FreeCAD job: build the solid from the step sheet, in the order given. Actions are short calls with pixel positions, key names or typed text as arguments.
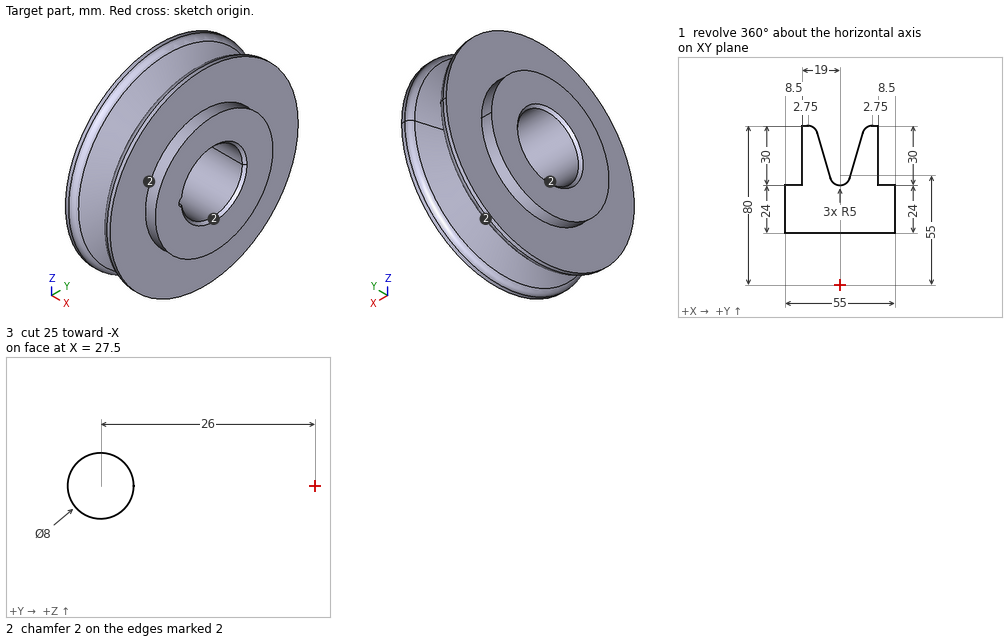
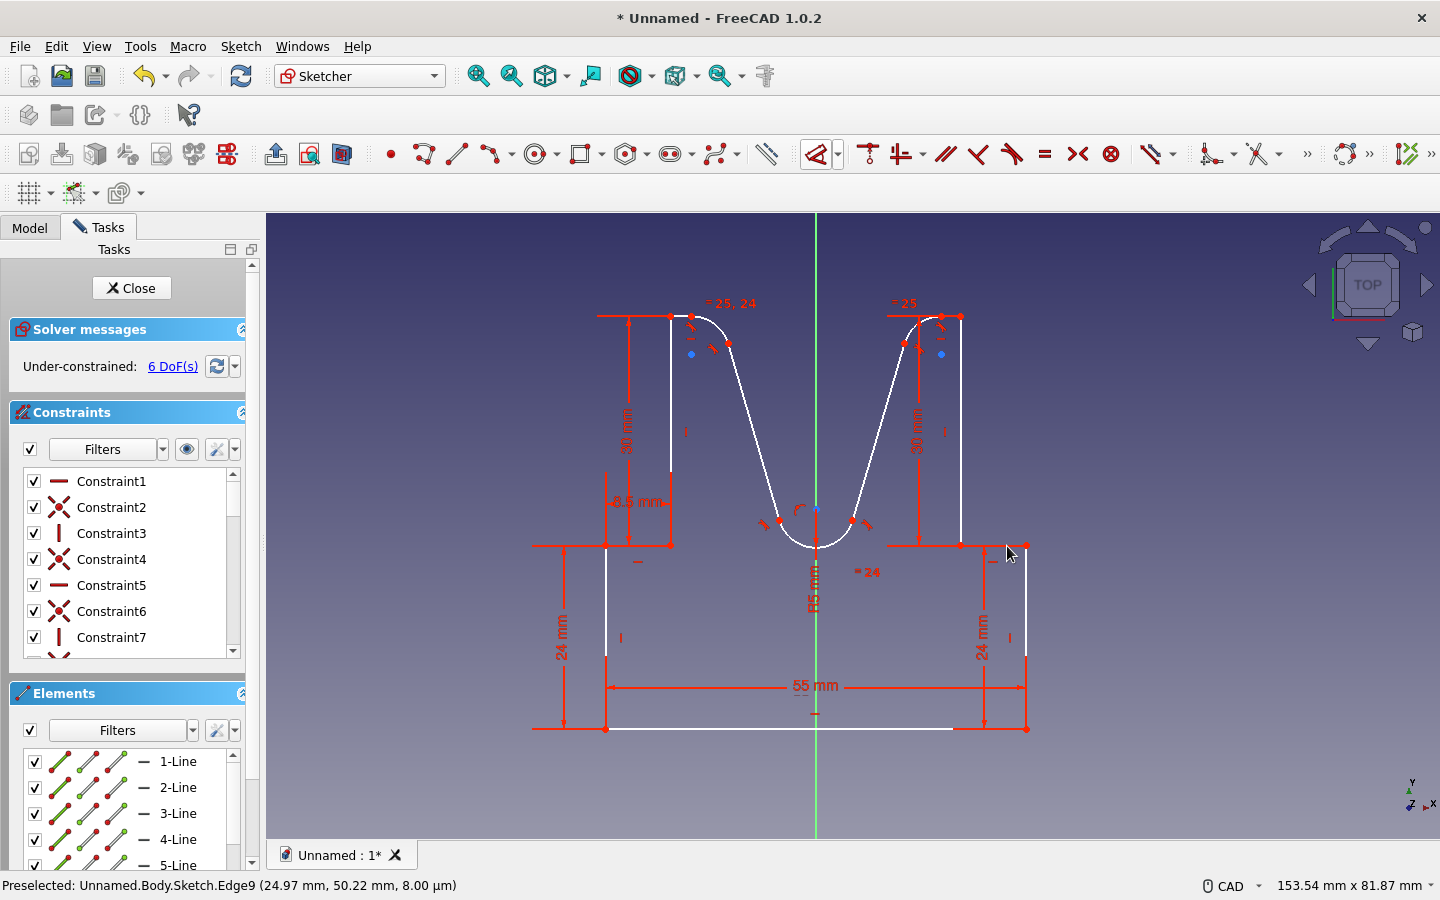
key(l)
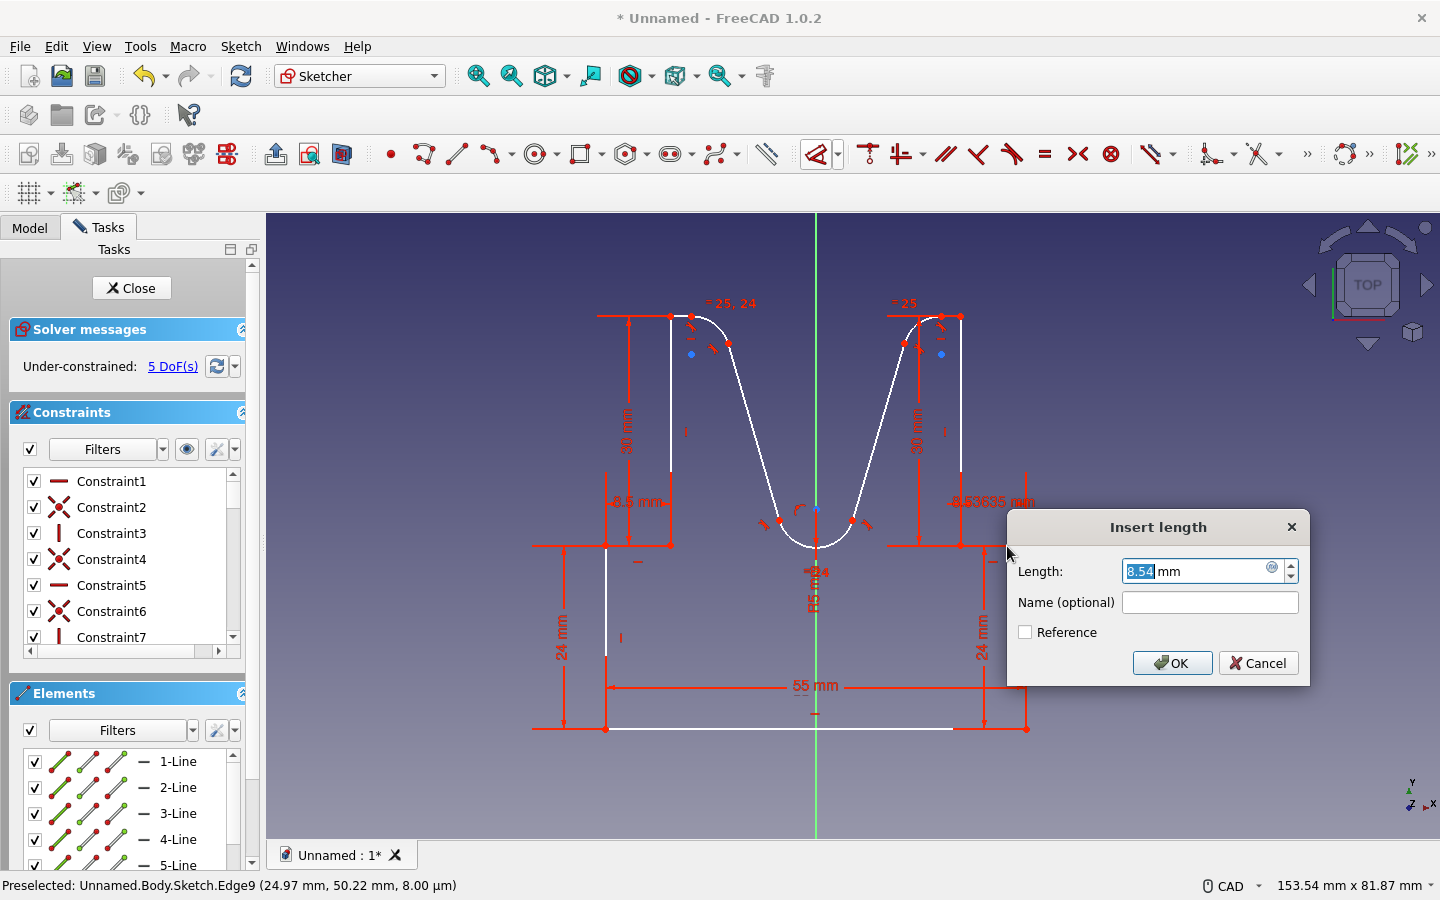
text(8.5)
key(Return)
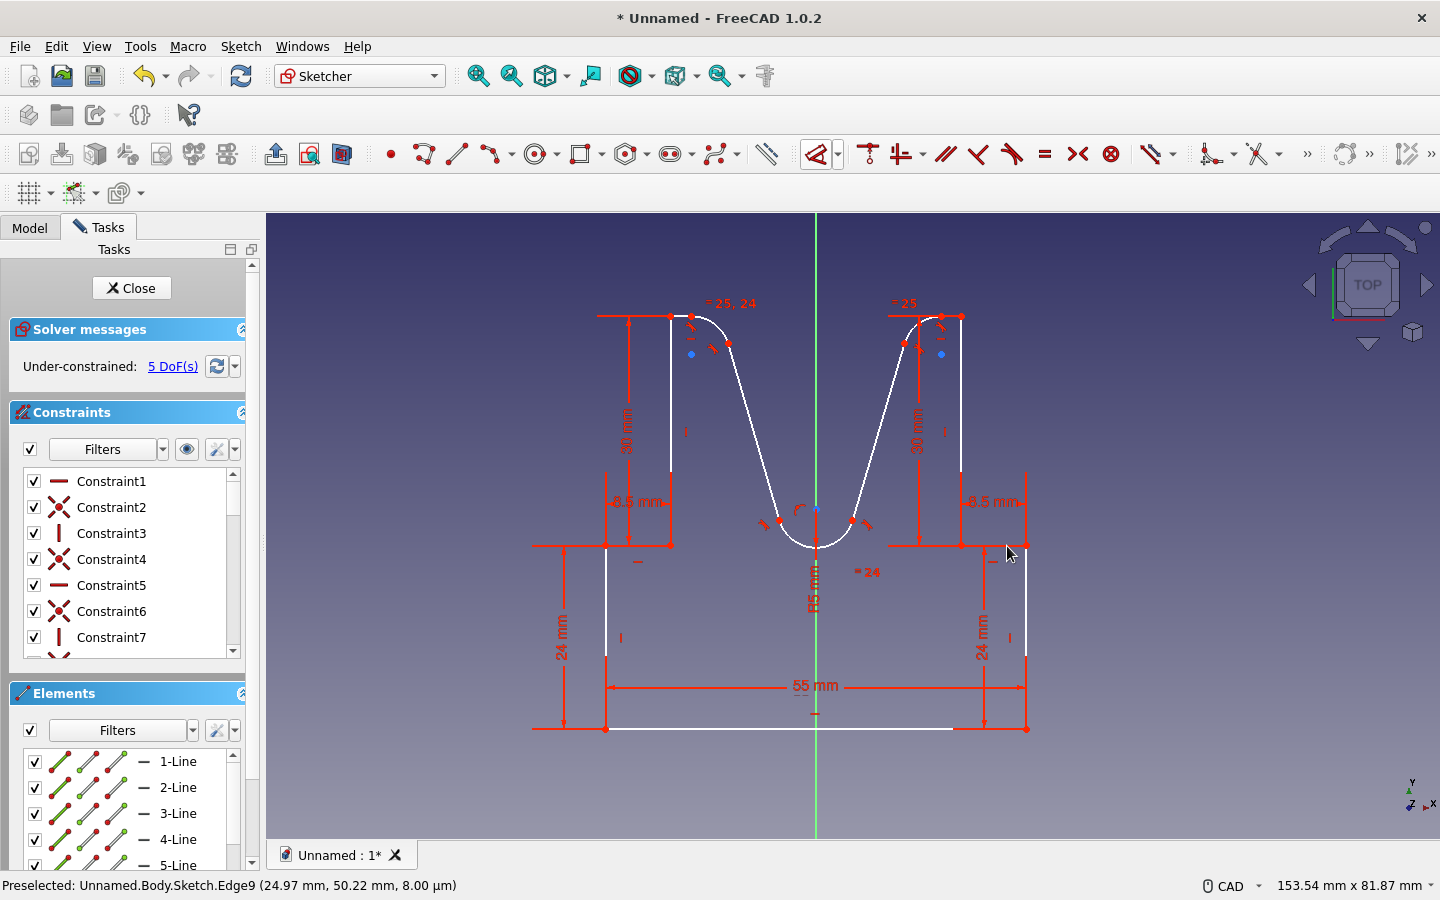
click(691, 316)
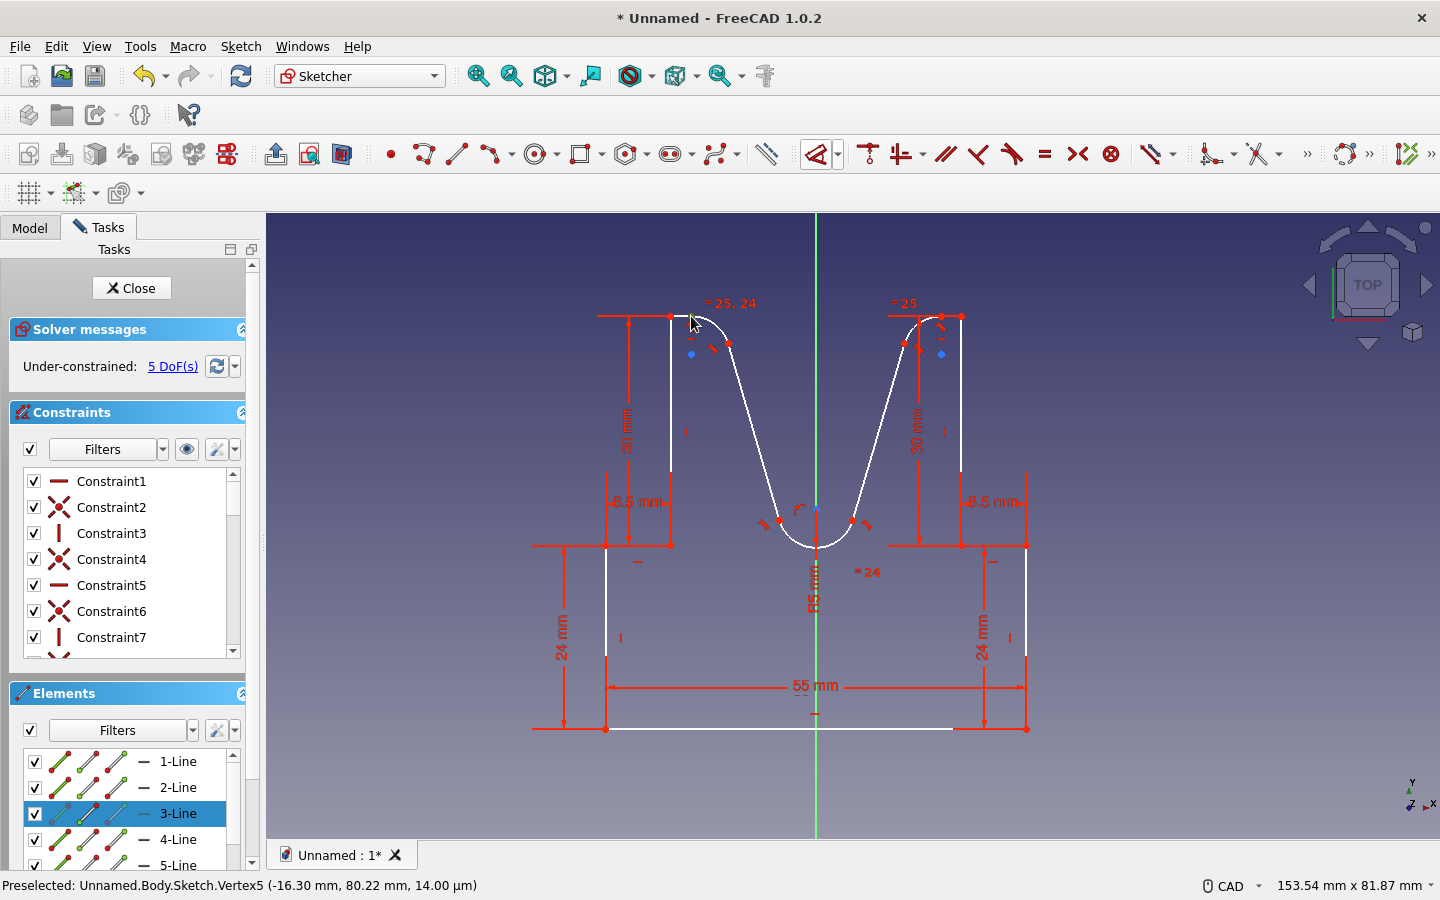
key(i)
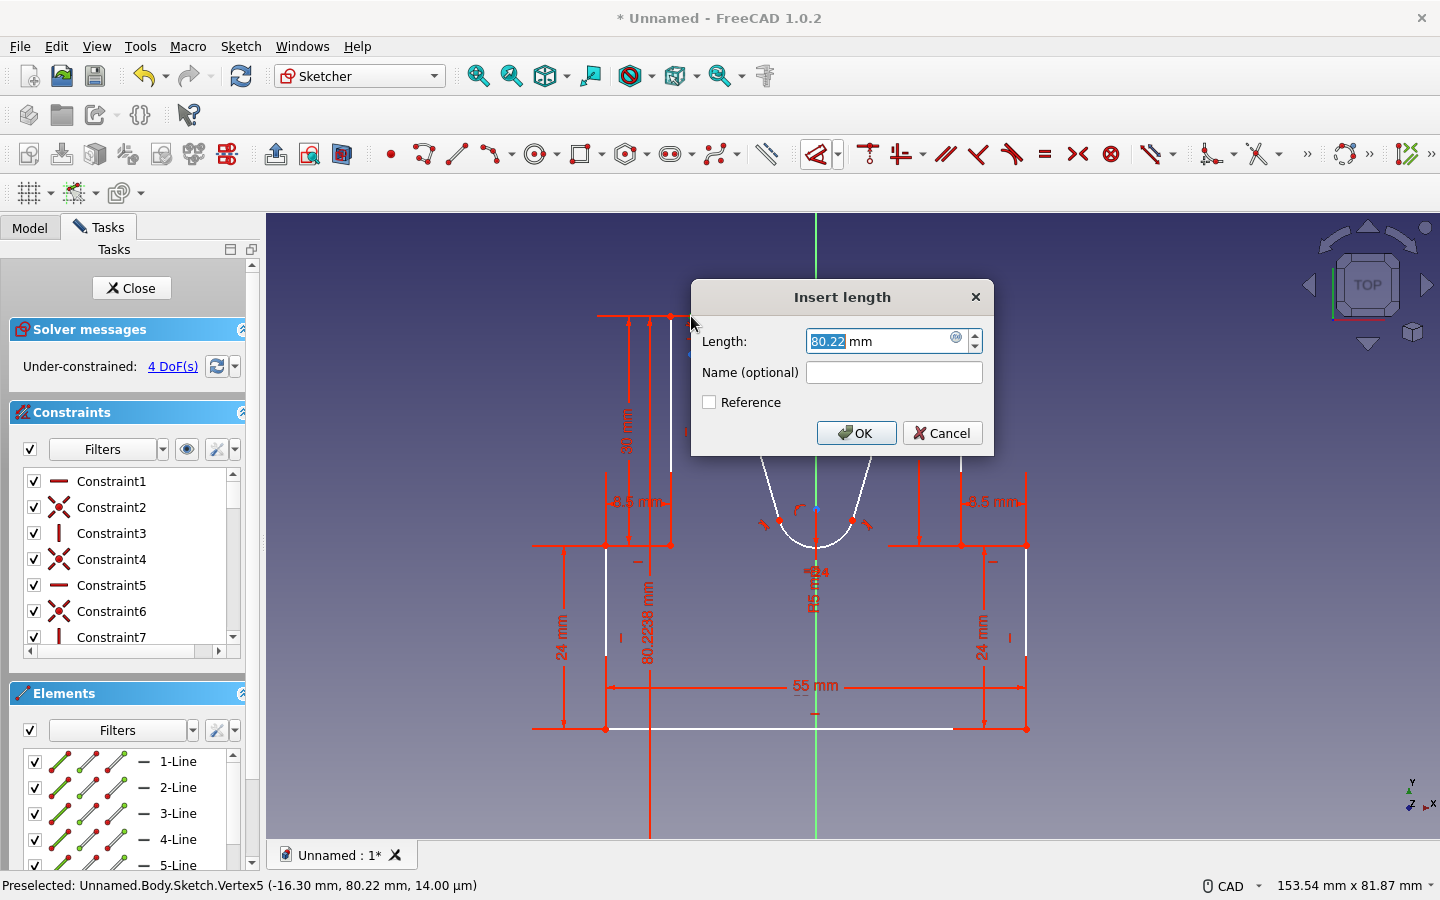
text(80)
key(Return)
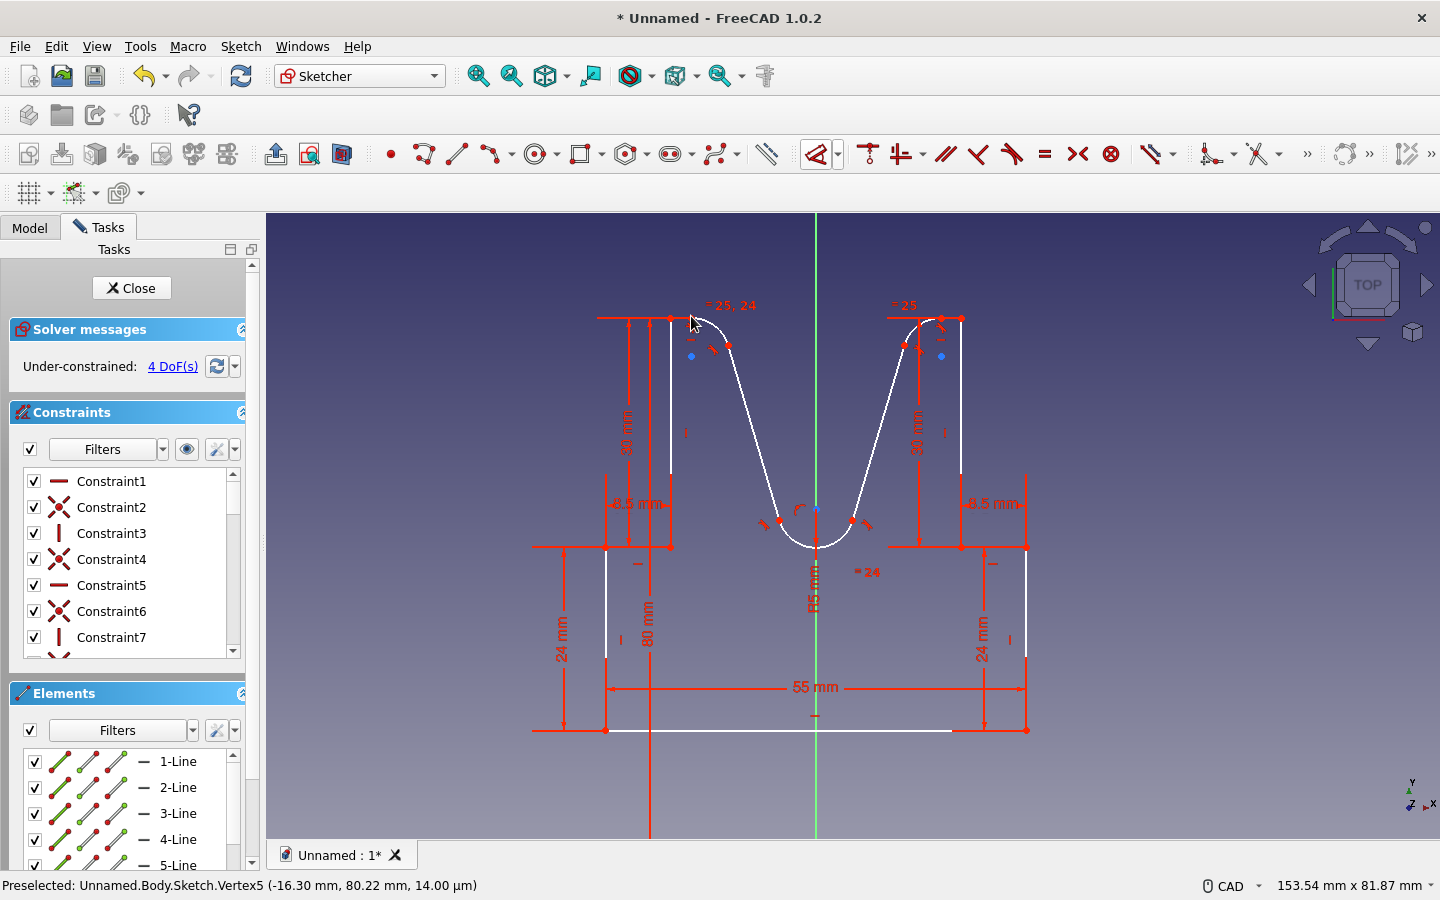
click(671, 318)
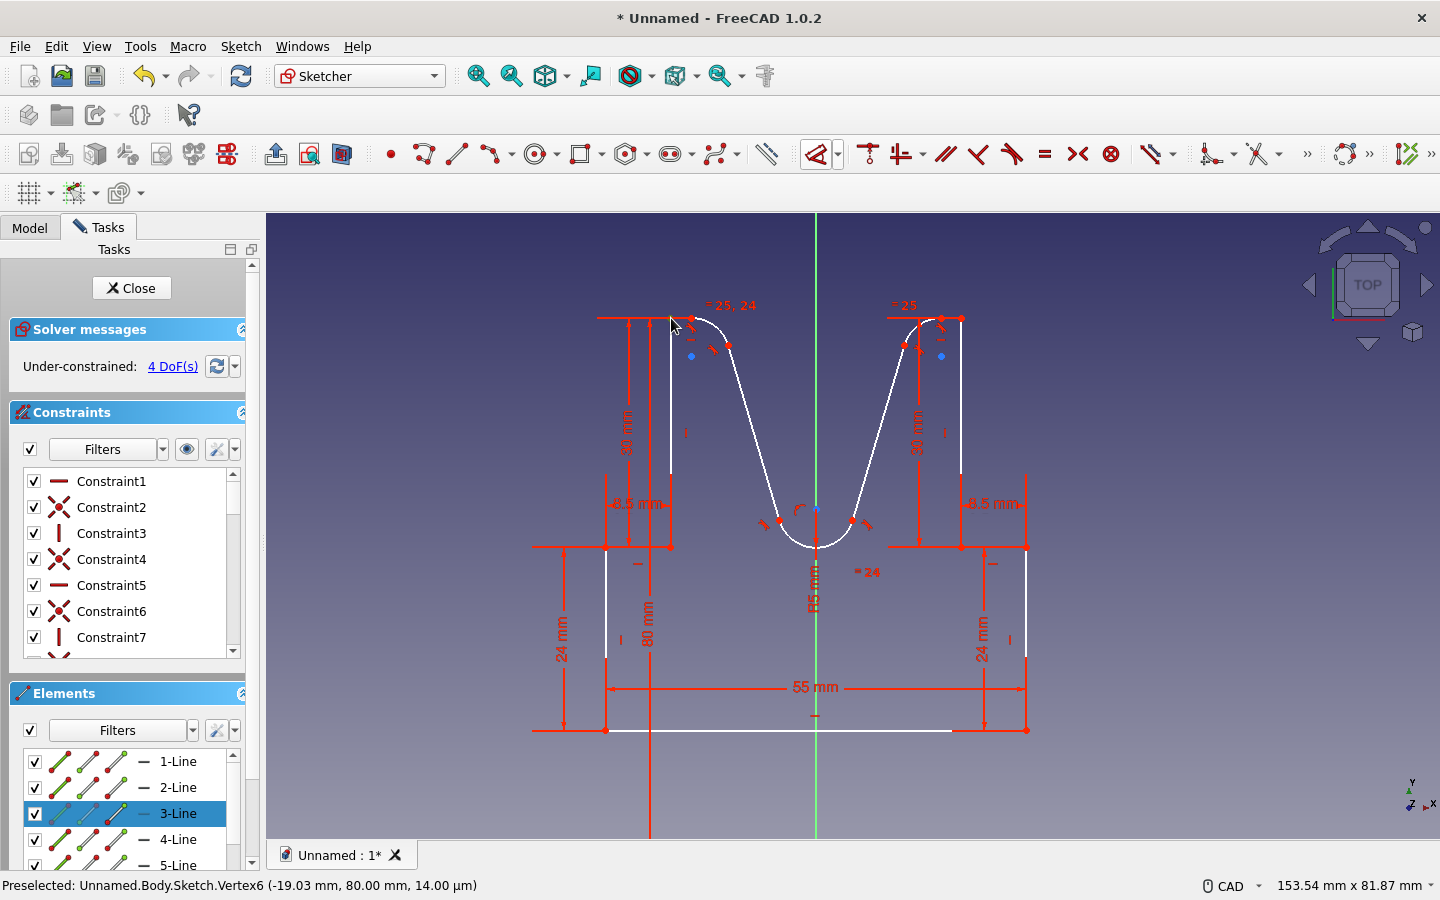
key(l)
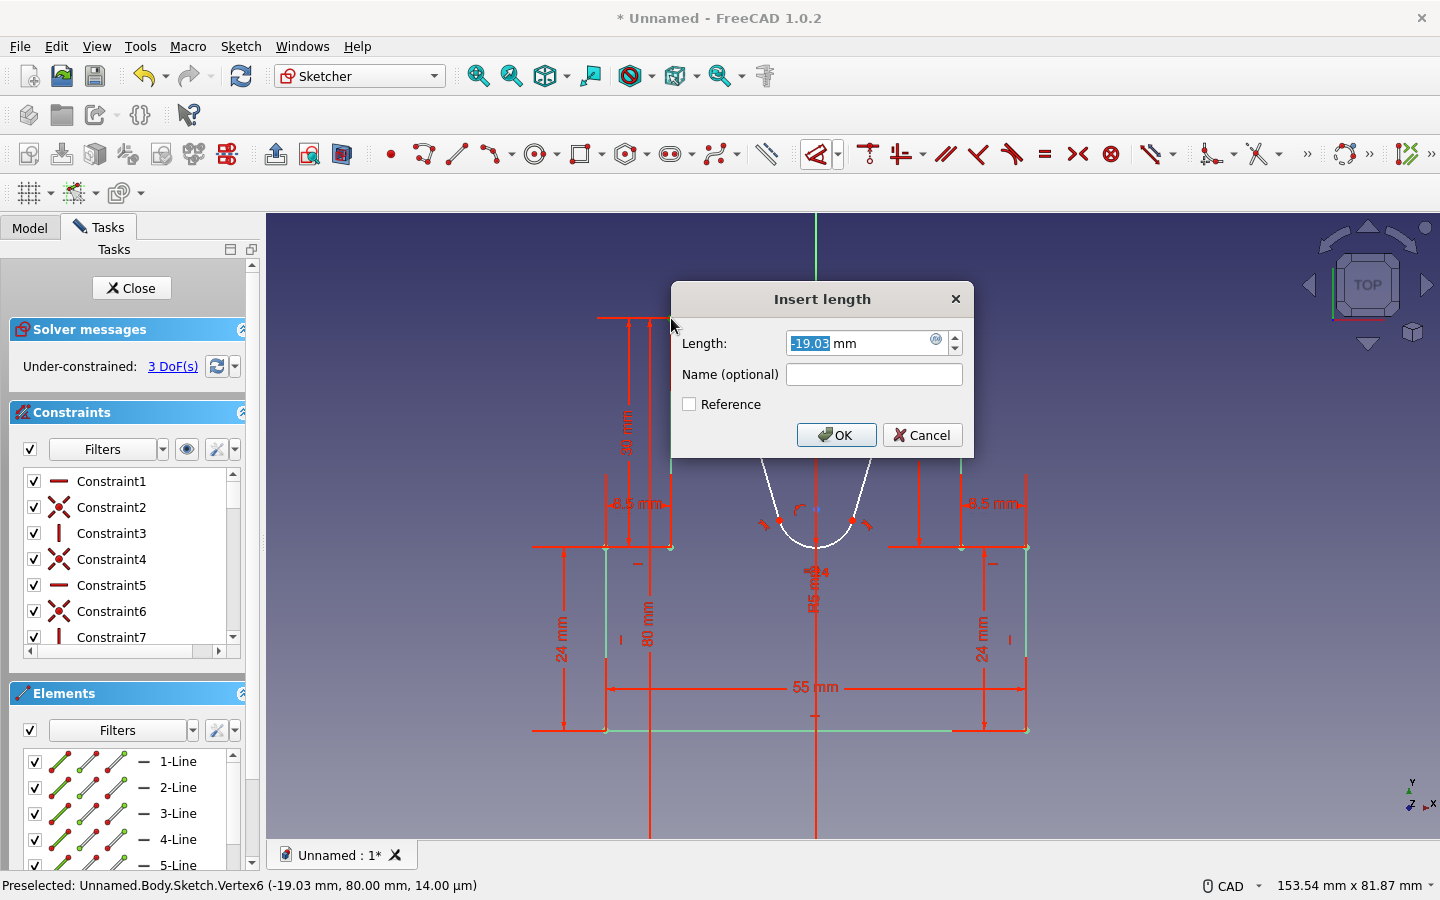
text(-19)
key(Return)